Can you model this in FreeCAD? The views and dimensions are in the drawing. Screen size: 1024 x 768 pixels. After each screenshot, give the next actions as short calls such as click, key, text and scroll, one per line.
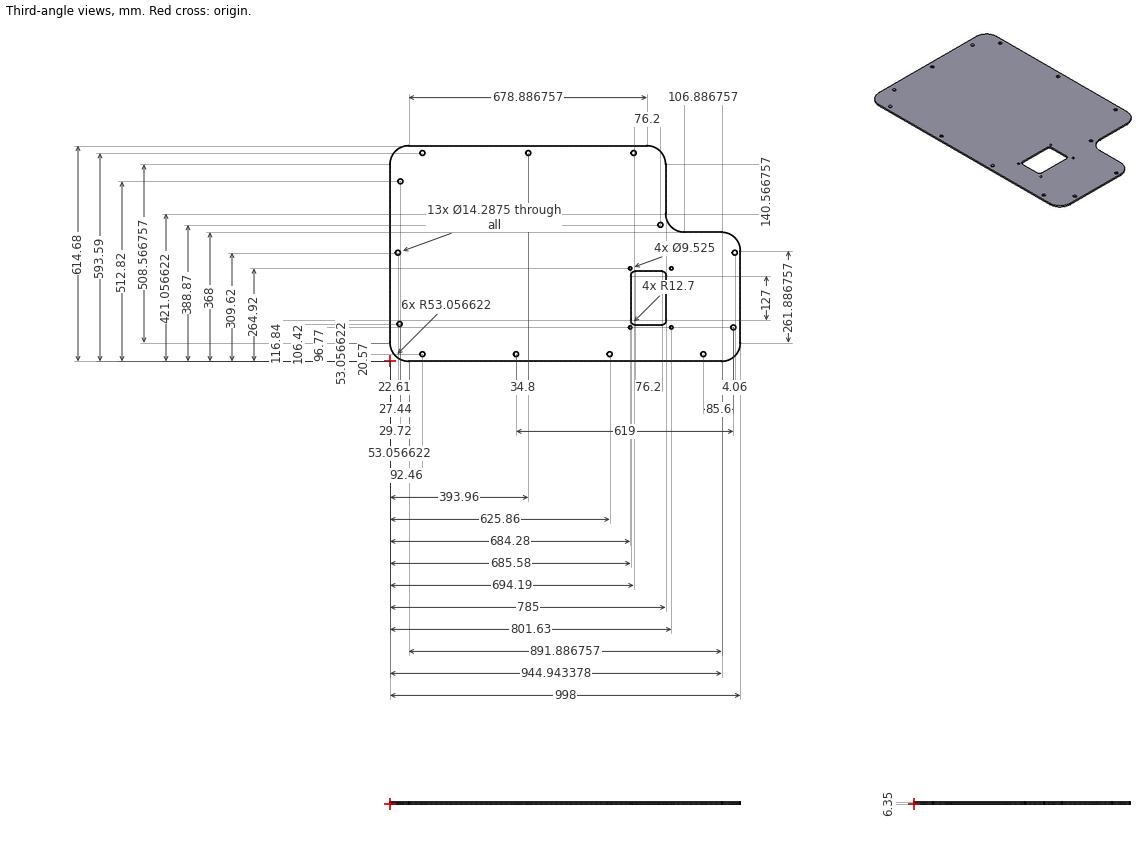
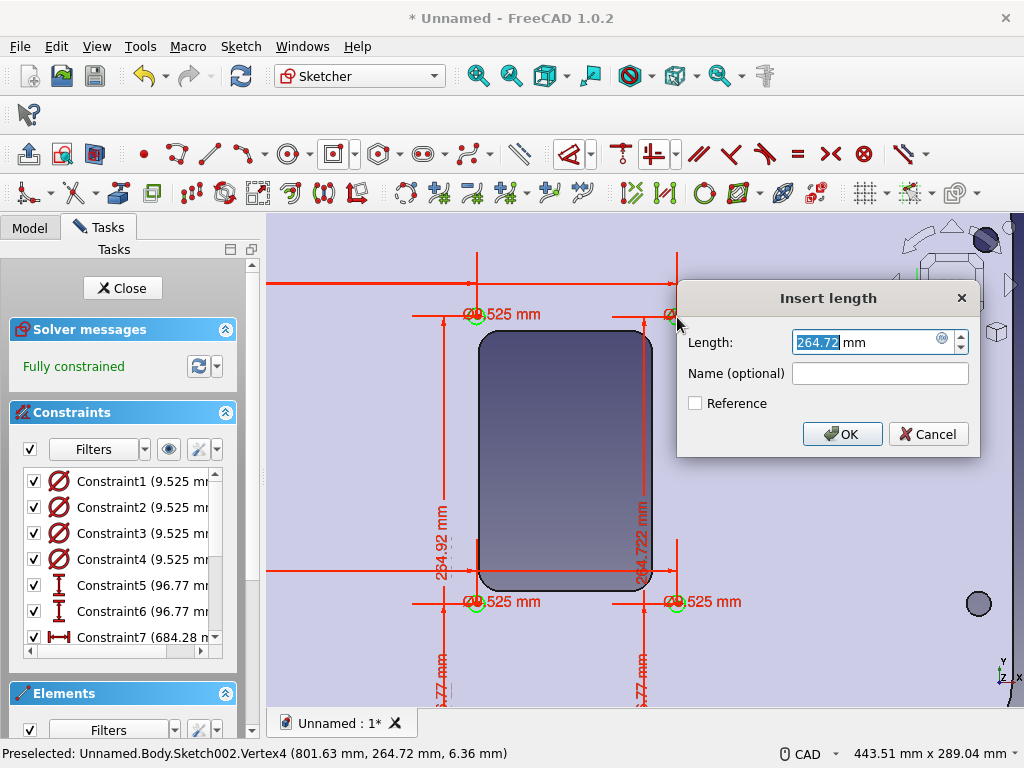
text(264.92)
key(Return)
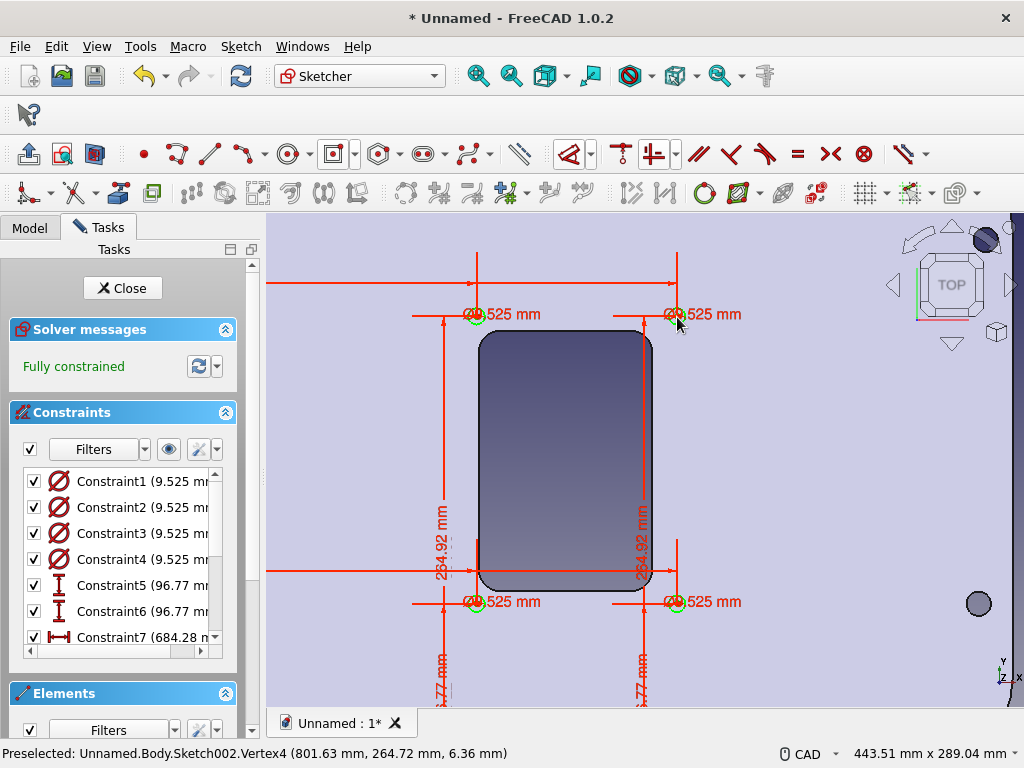
click(123, 288)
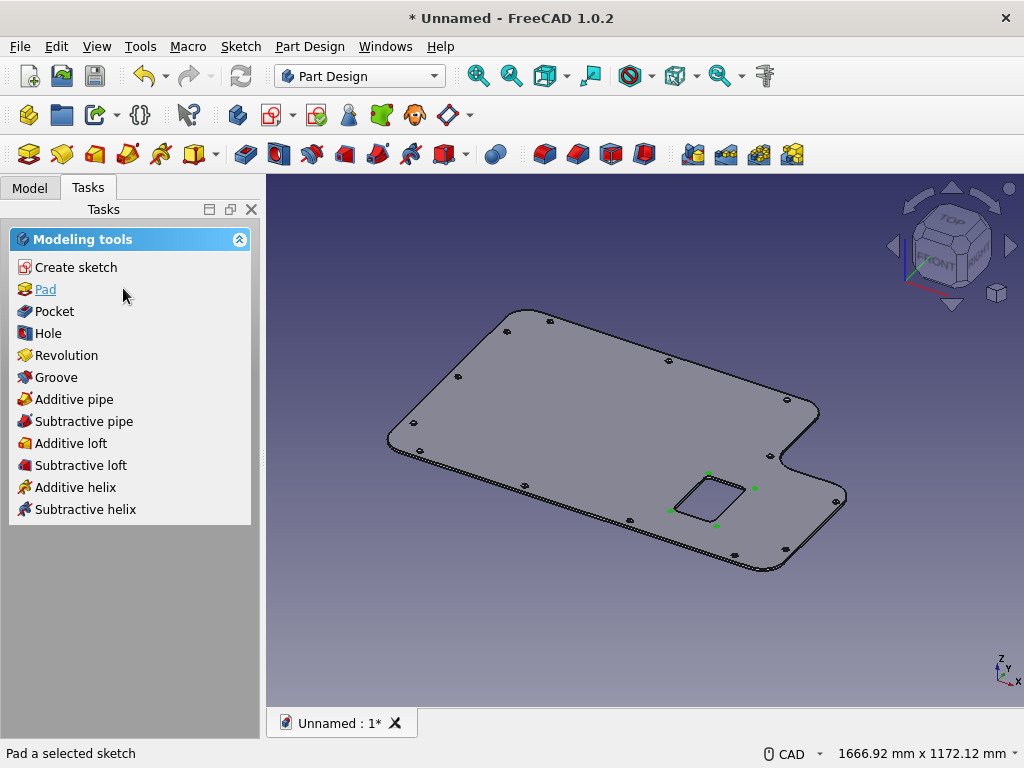
click(246, 154)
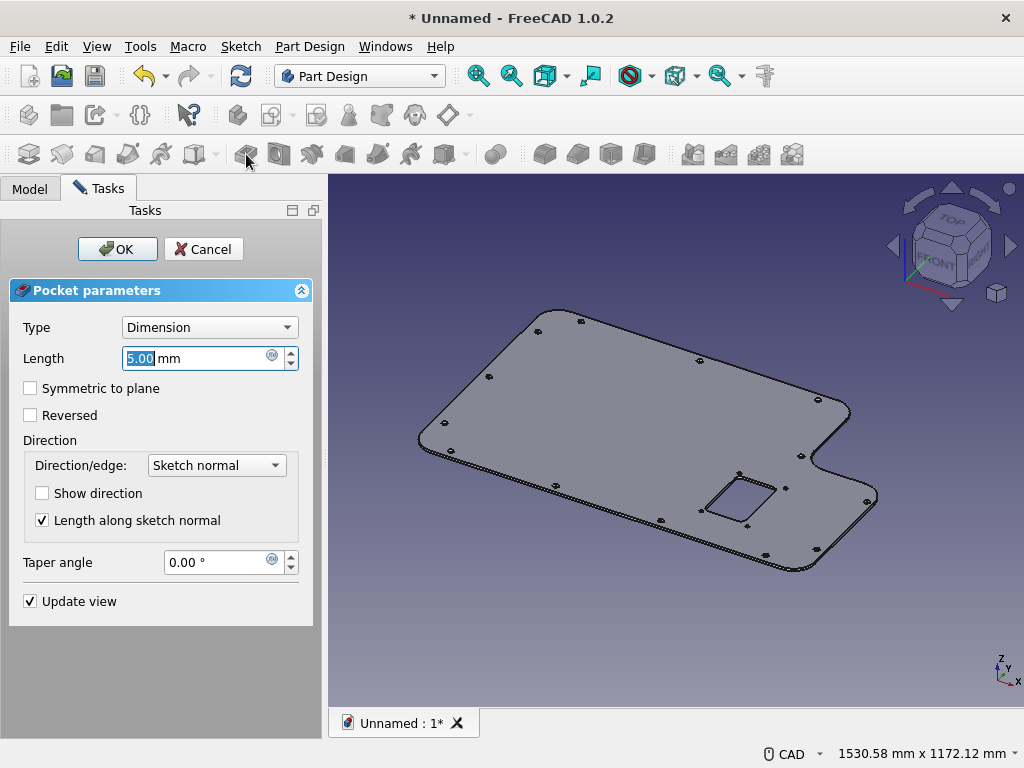
click(210, 328)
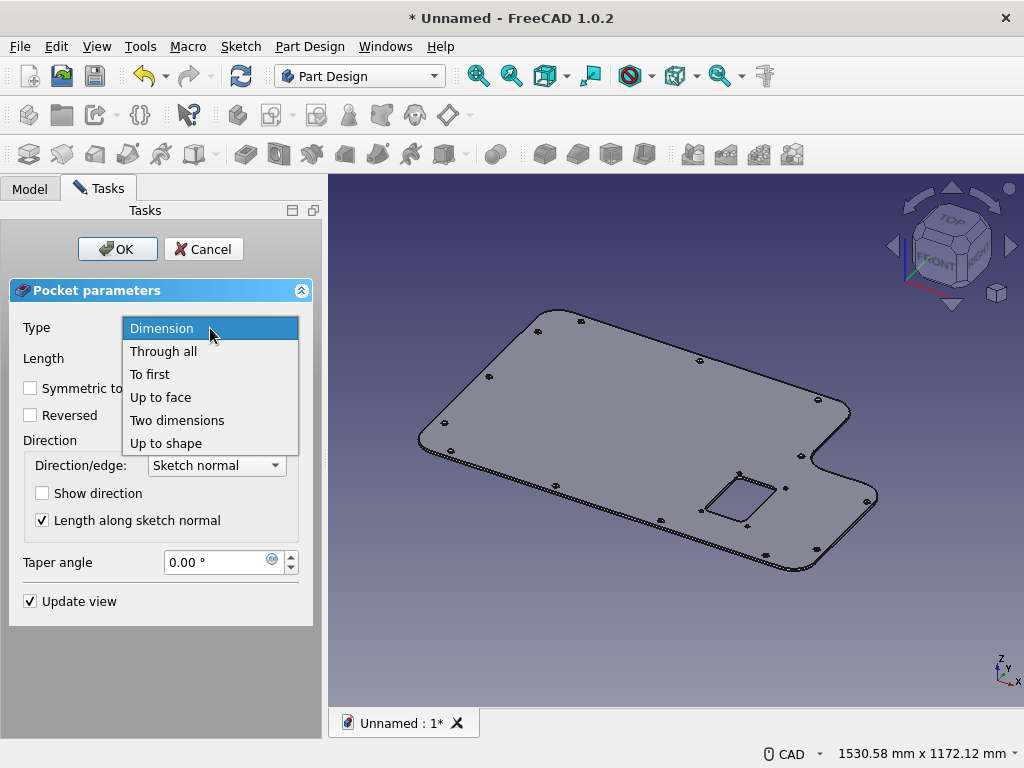
click(208, 352)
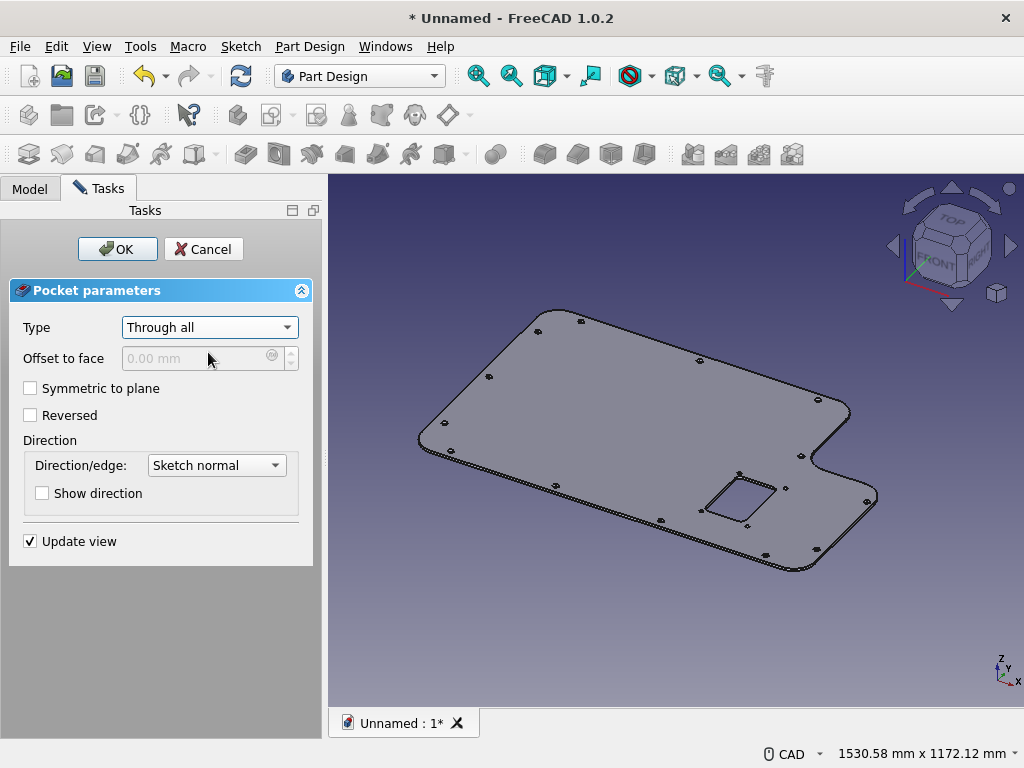
click(118, 249)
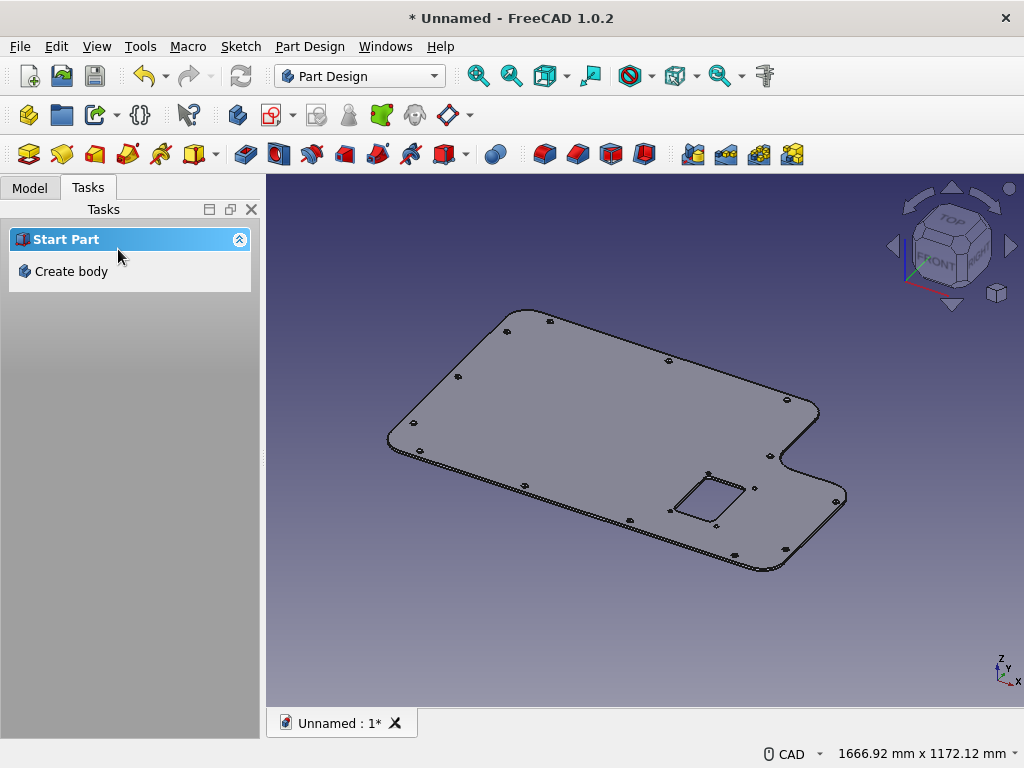
key(0)